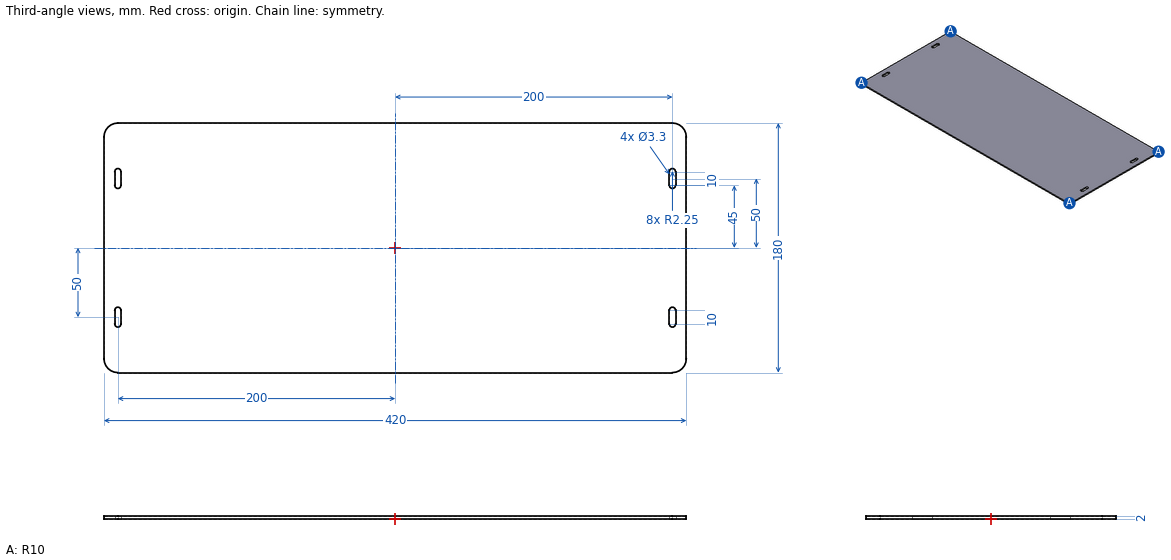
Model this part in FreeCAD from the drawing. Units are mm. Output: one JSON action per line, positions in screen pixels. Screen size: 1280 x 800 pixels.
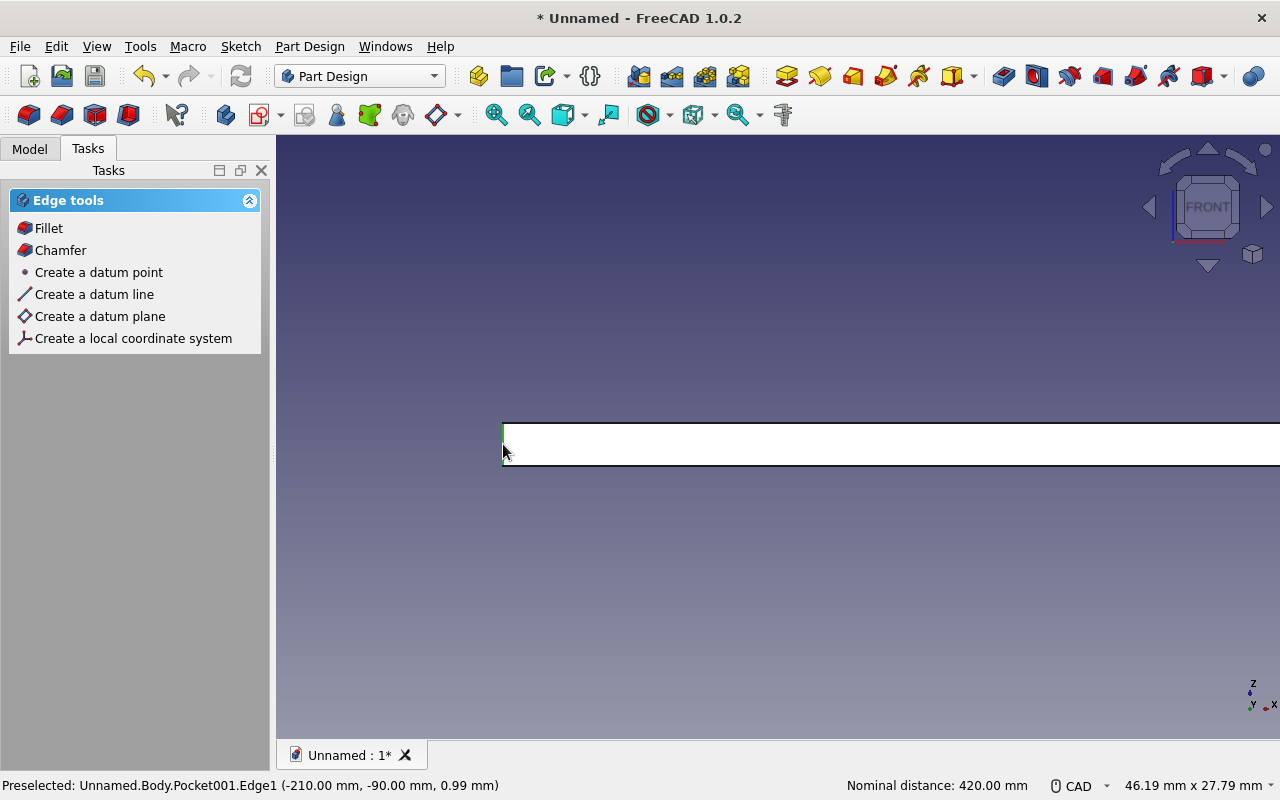
{"action": "key", "text": "v f"}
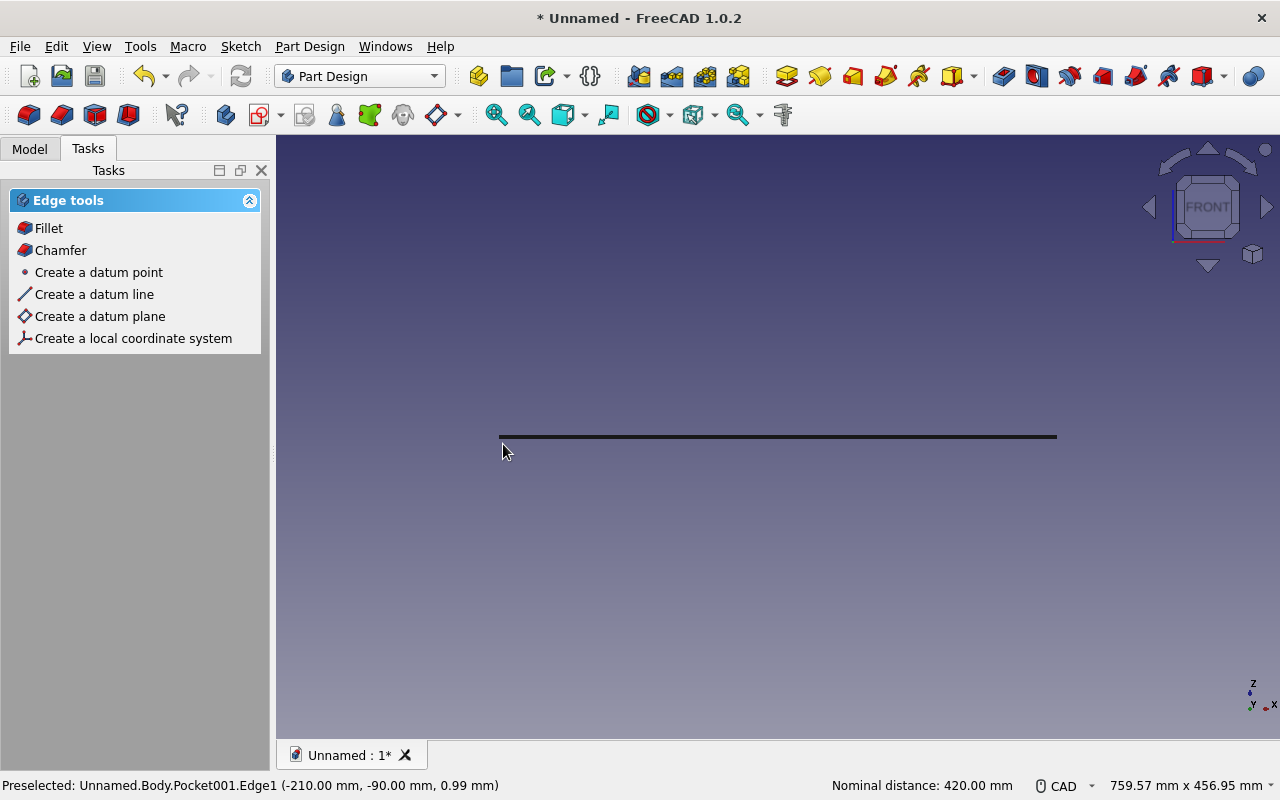
{"action": "key", "text": "3"}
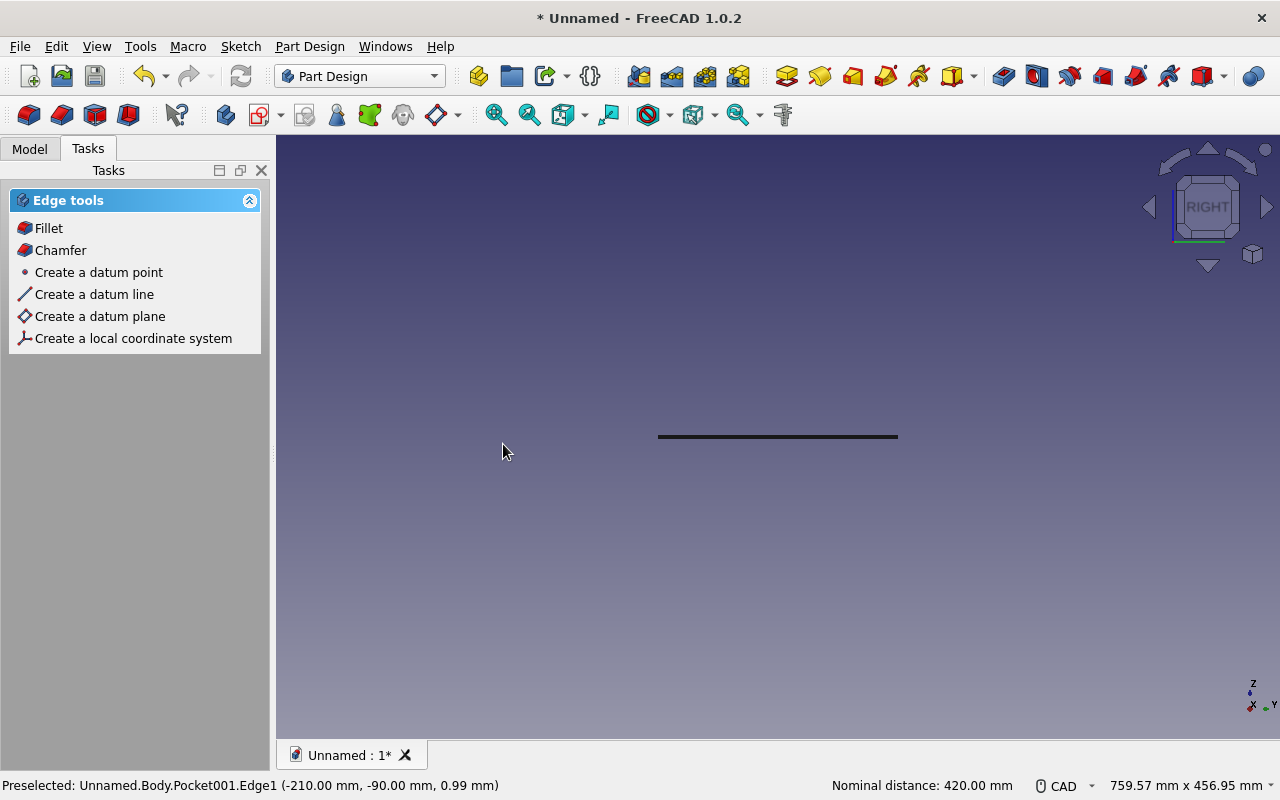
{"action": "left_click", "coordinate": [497, 116]}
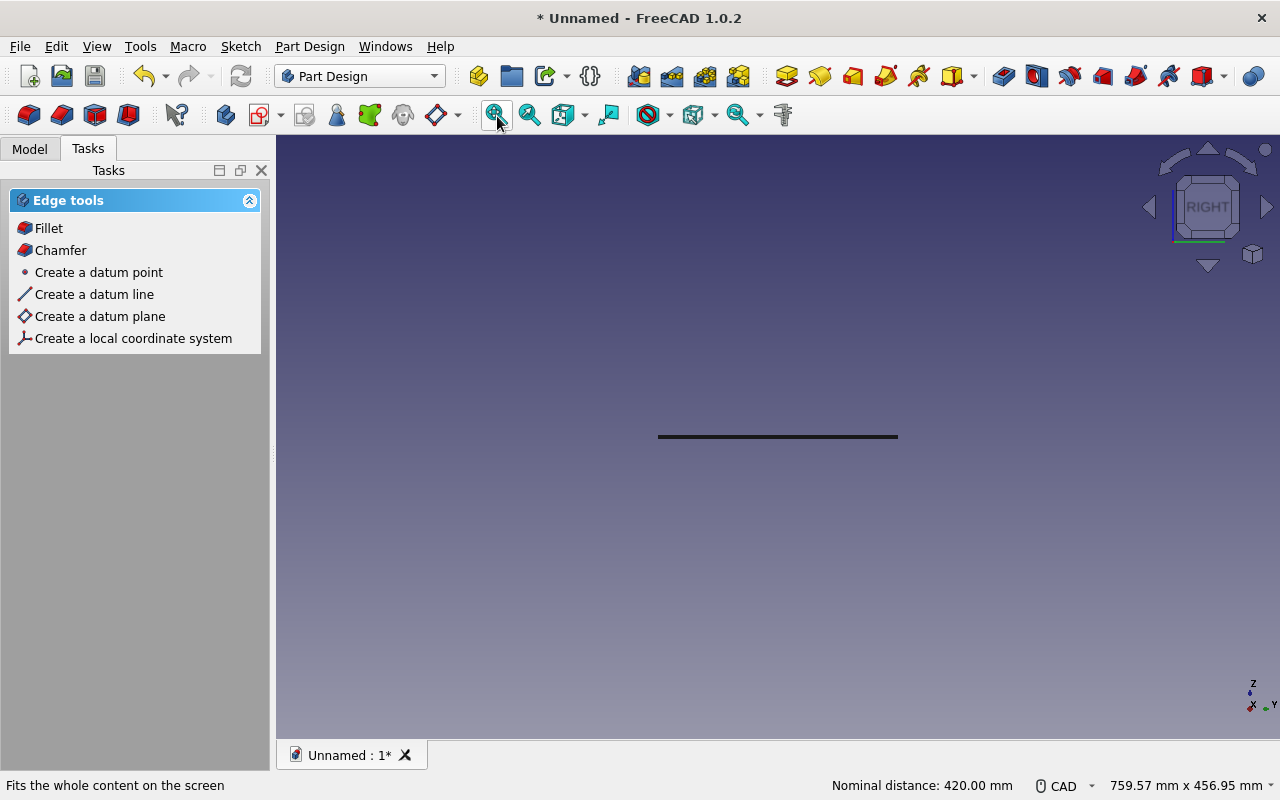
{"action": "scroll", "coordinate": [897, 436], "scroll_direction": "up", "scroll_amount": 14}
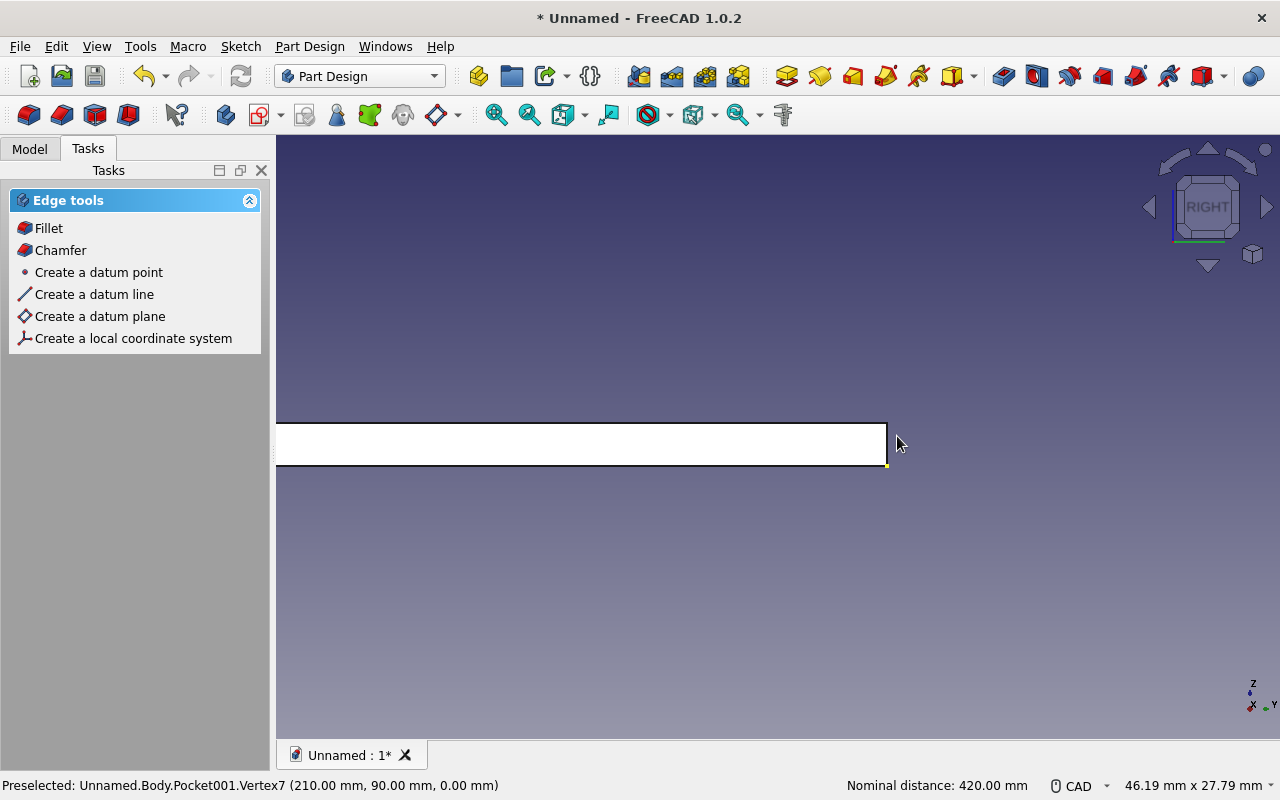
{"action": "left_click", "coordinate": [887, 444], "text": "ctrl"}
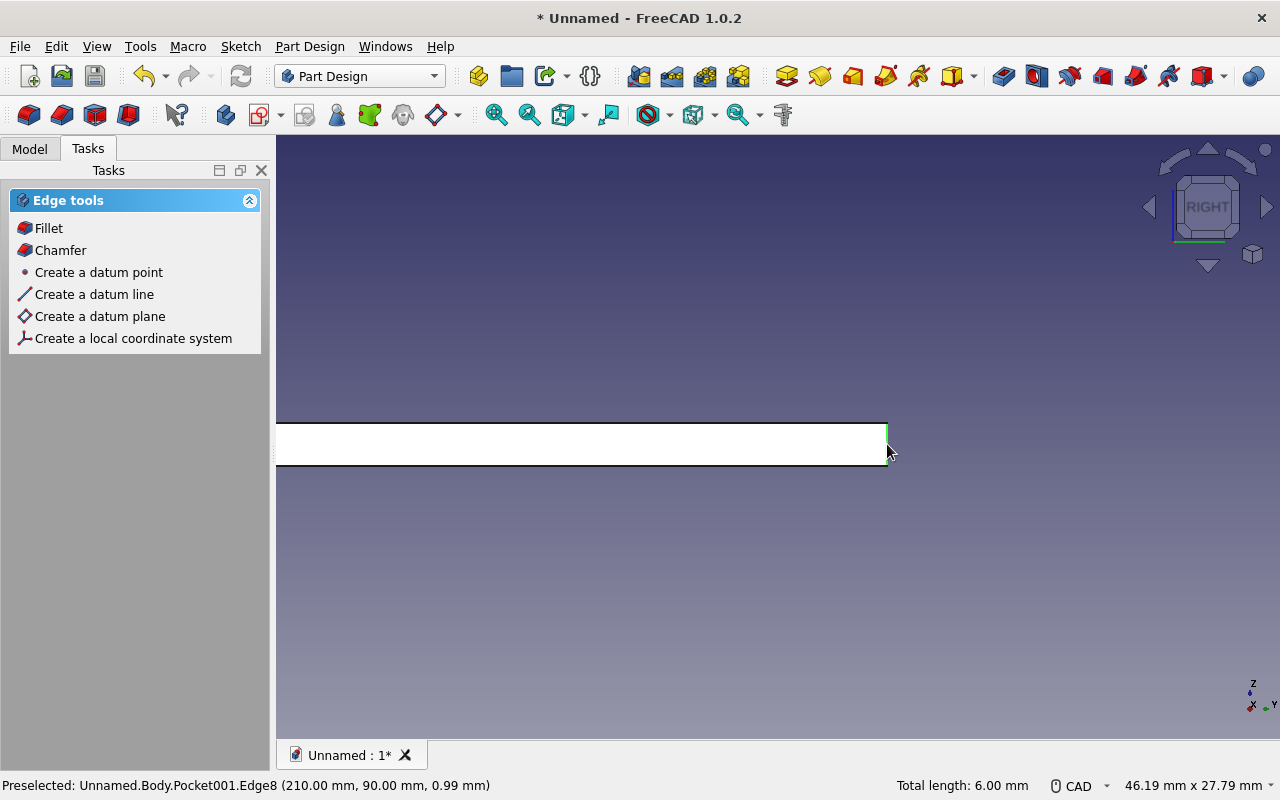
{"action": "key", "text": "v f"}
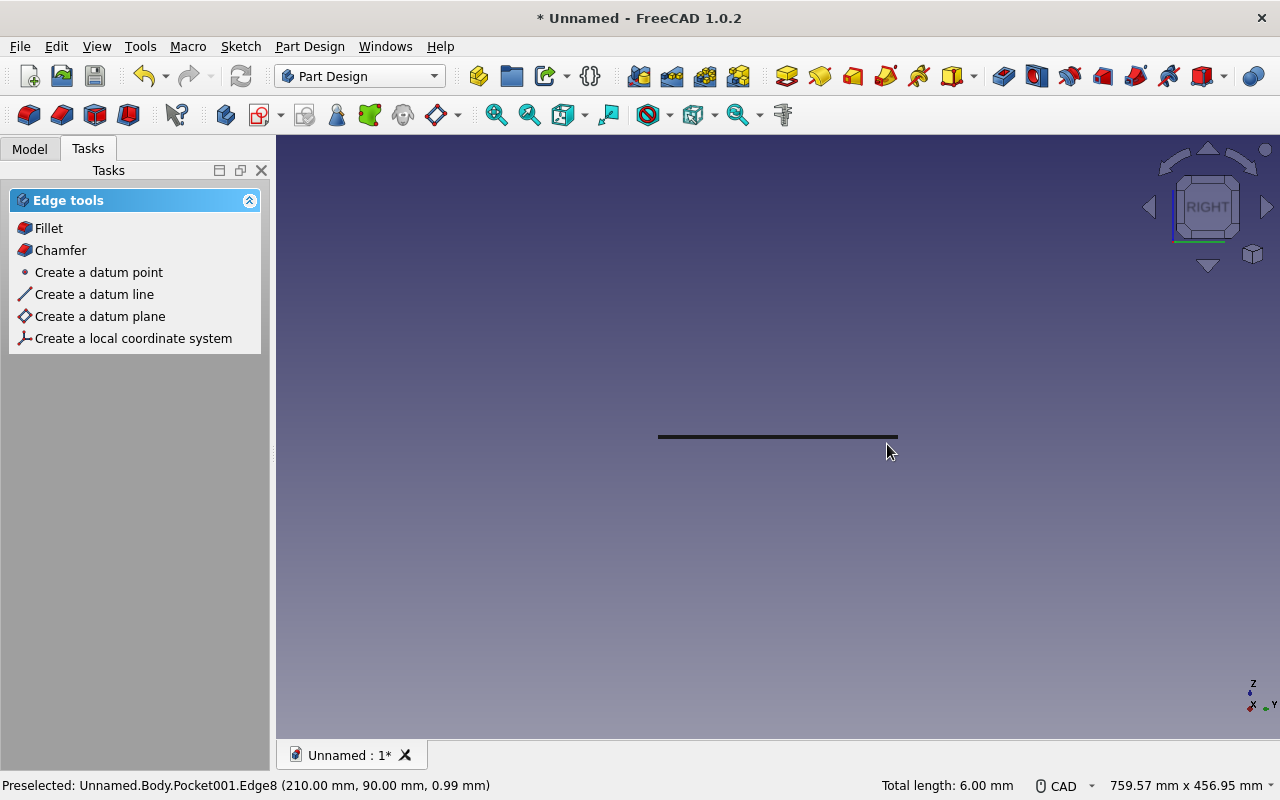
{"action": "key", "text": "5"}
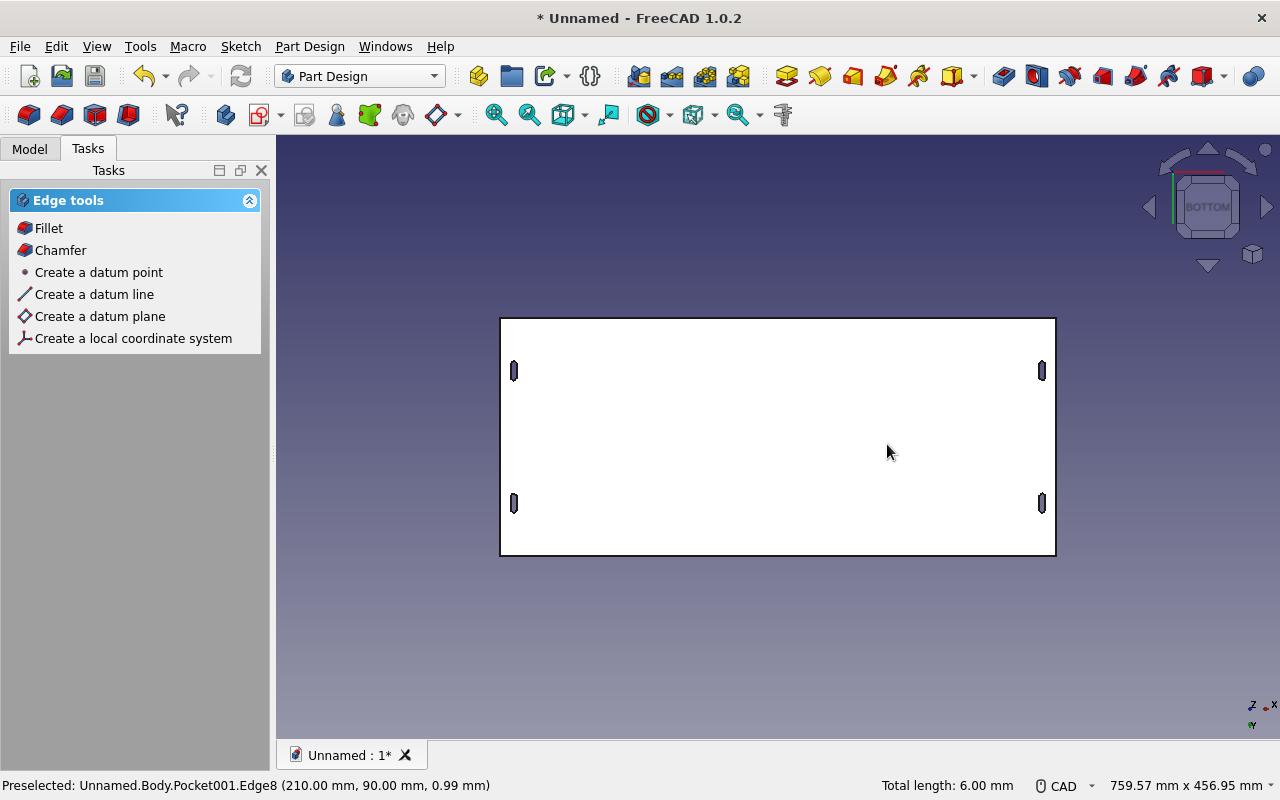
{"action": "scroll", "coordinate": [500, 555], "scroll_direction": "up", "scroll_amount": 14}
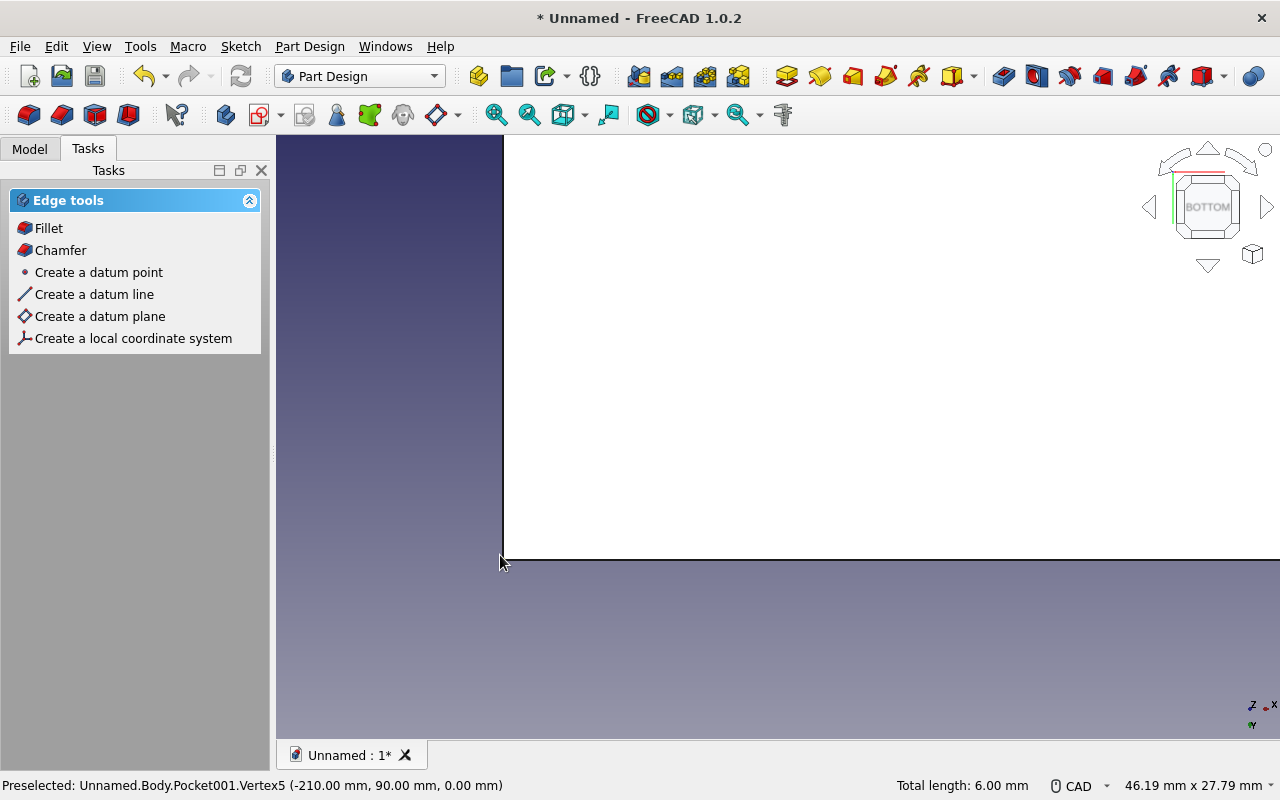
{"action": "key", "text": "v f"}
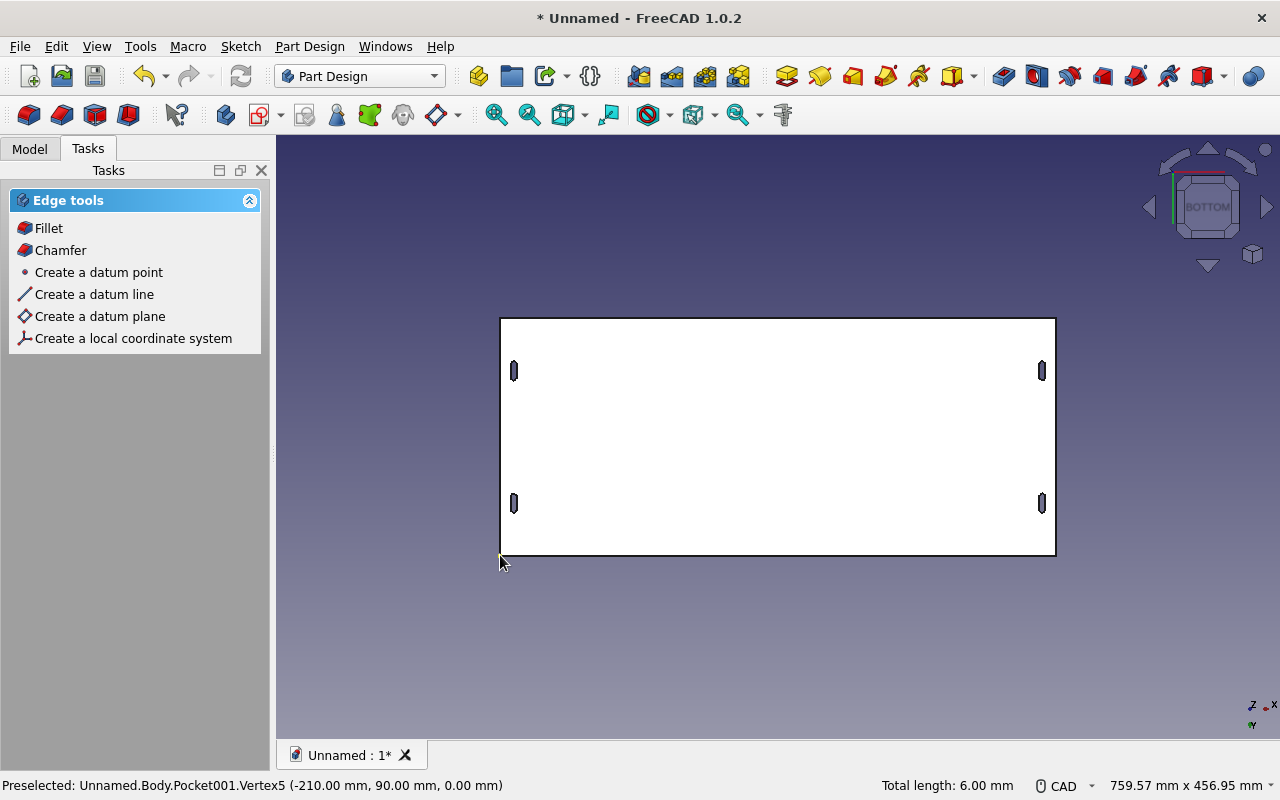
{"action": "key", "text": "4"}